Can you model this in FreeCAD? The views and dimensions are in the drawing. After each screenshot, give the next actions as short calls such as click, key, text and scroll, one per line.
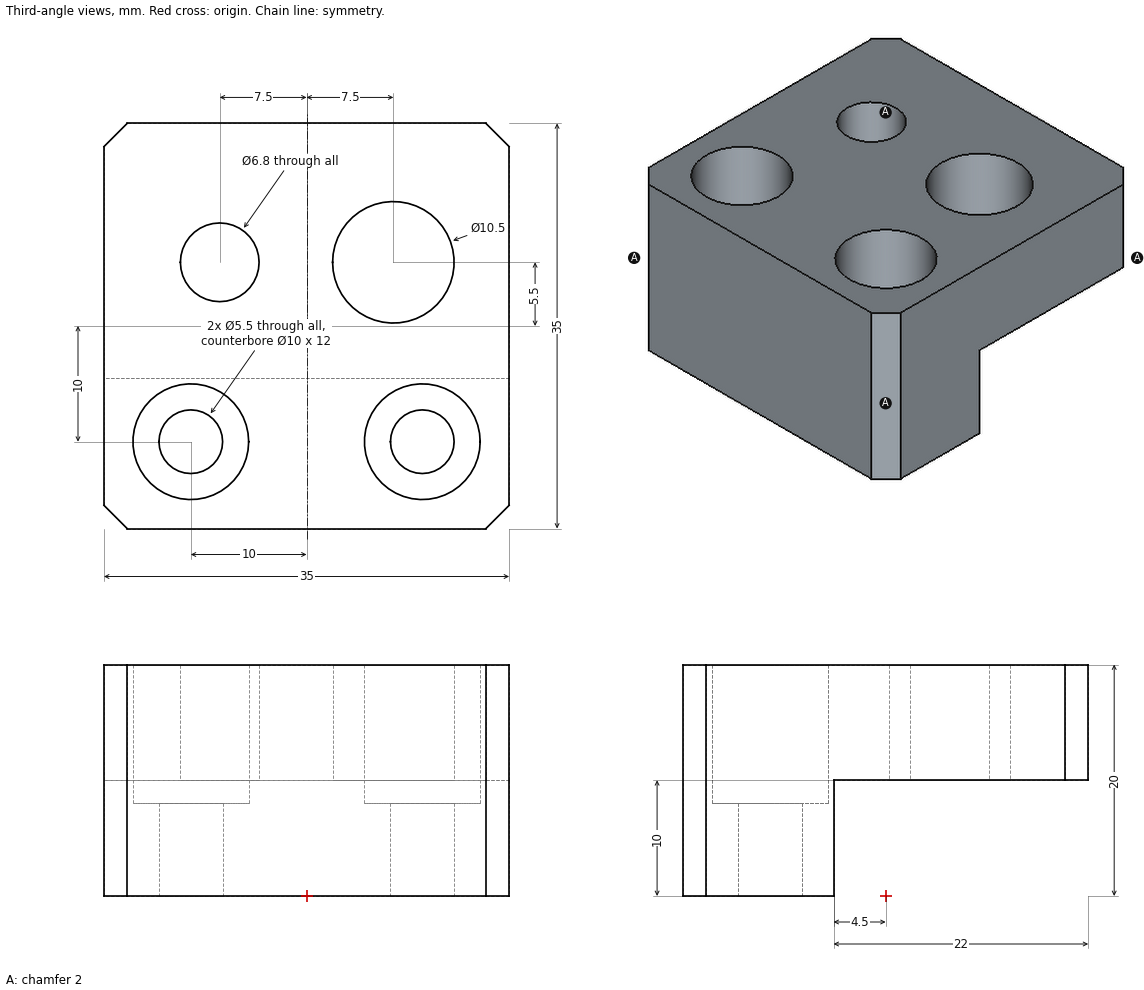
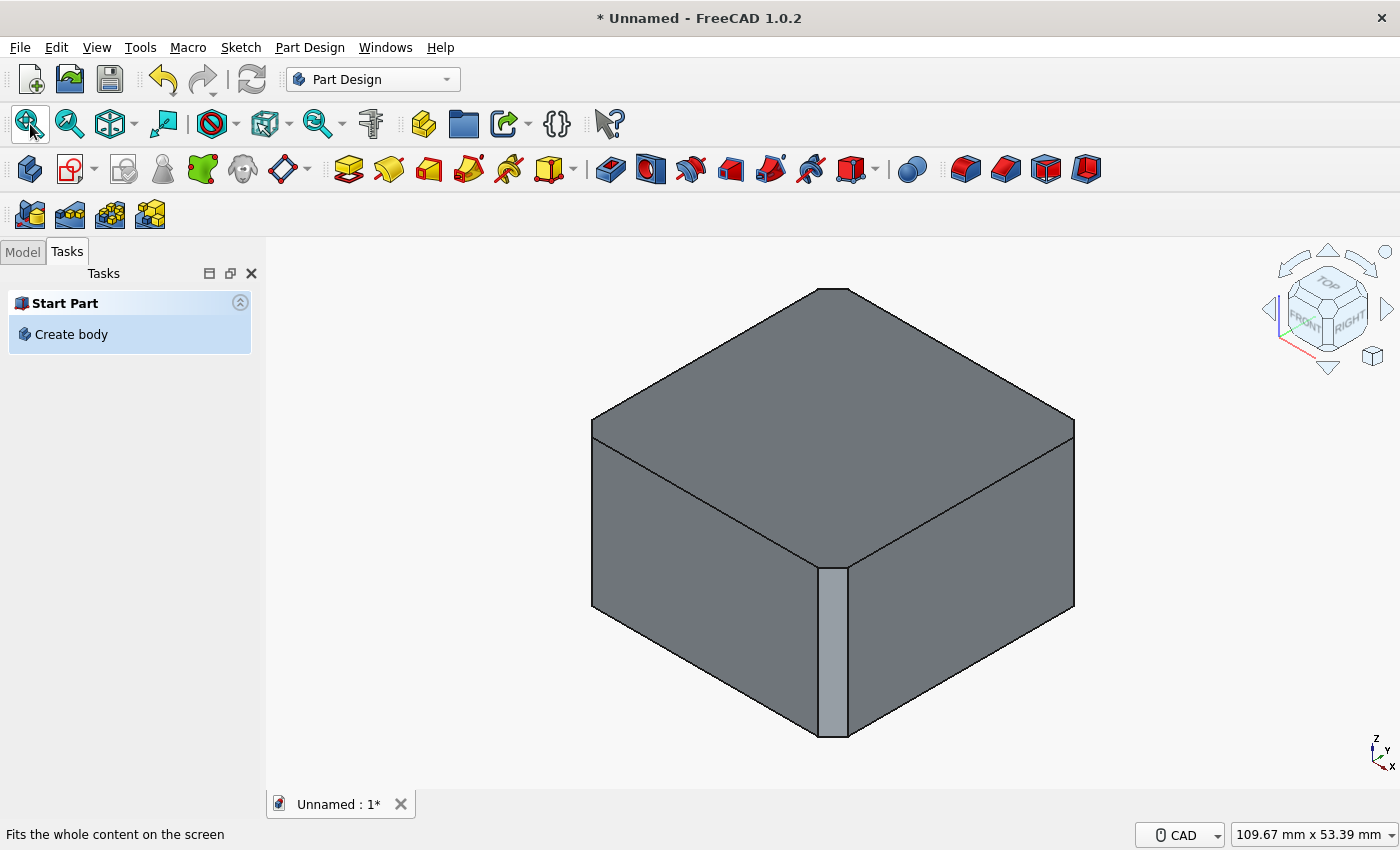
click(833, 428)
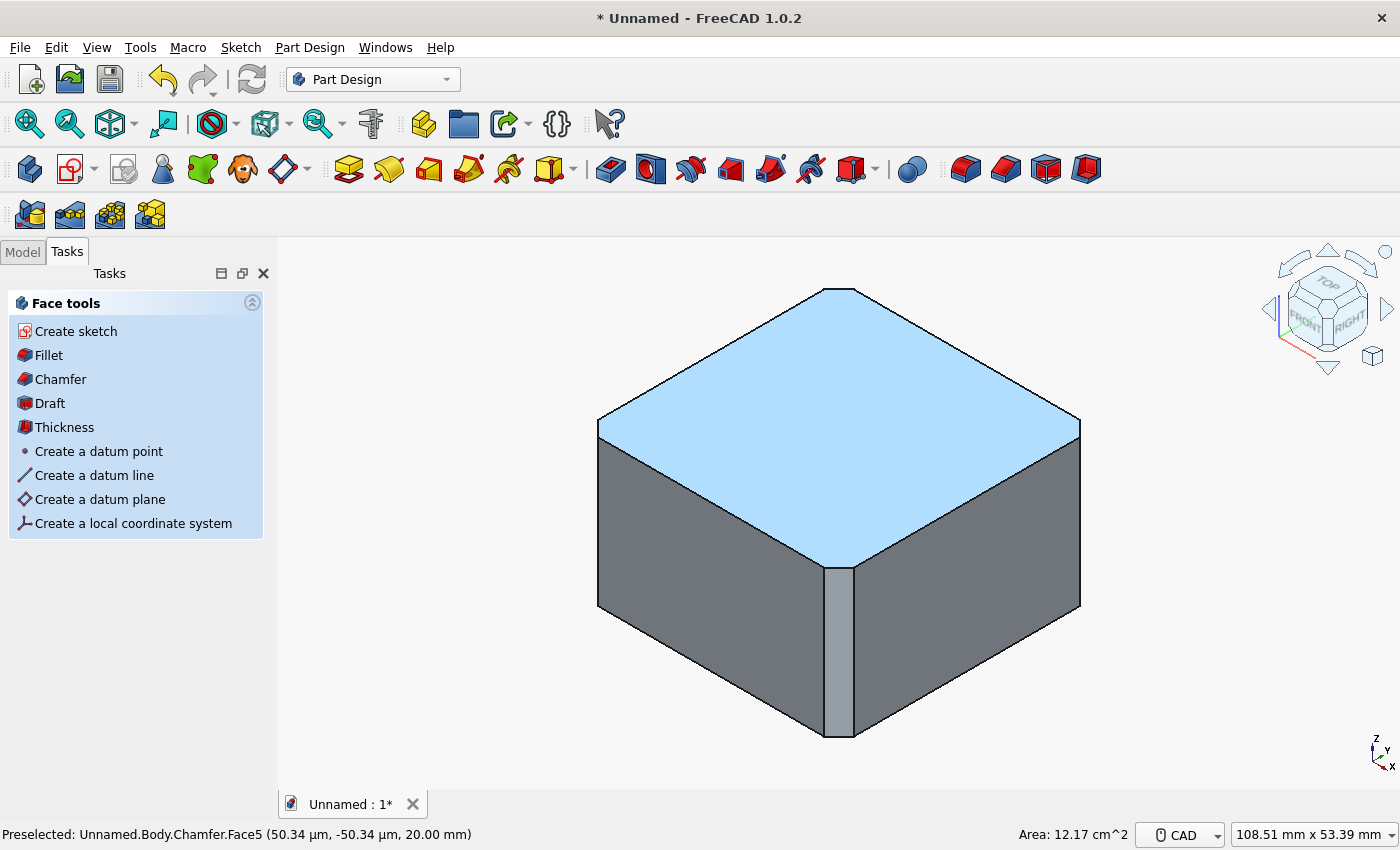
click(70, 170)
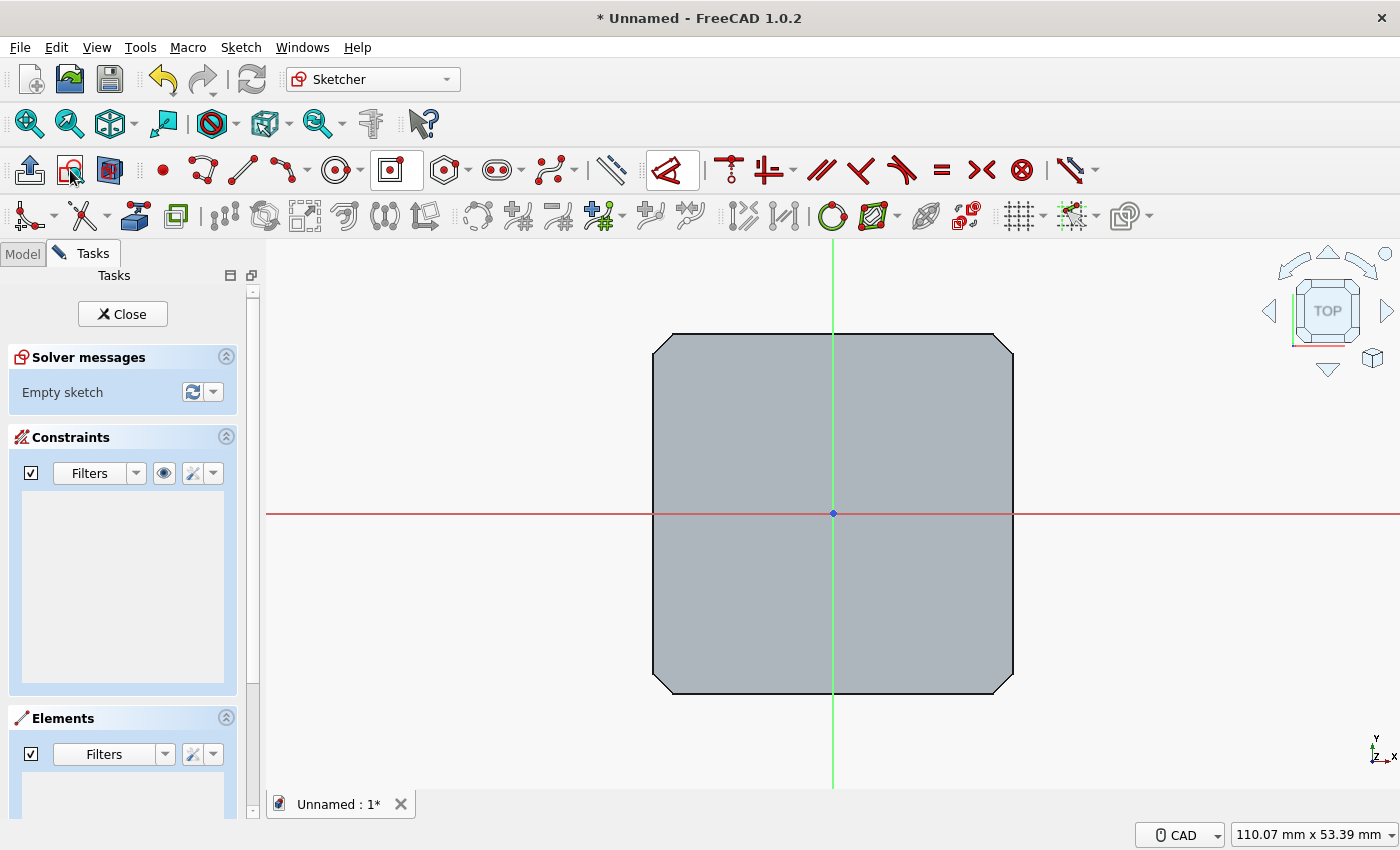
scroll(957, 435, up, 6)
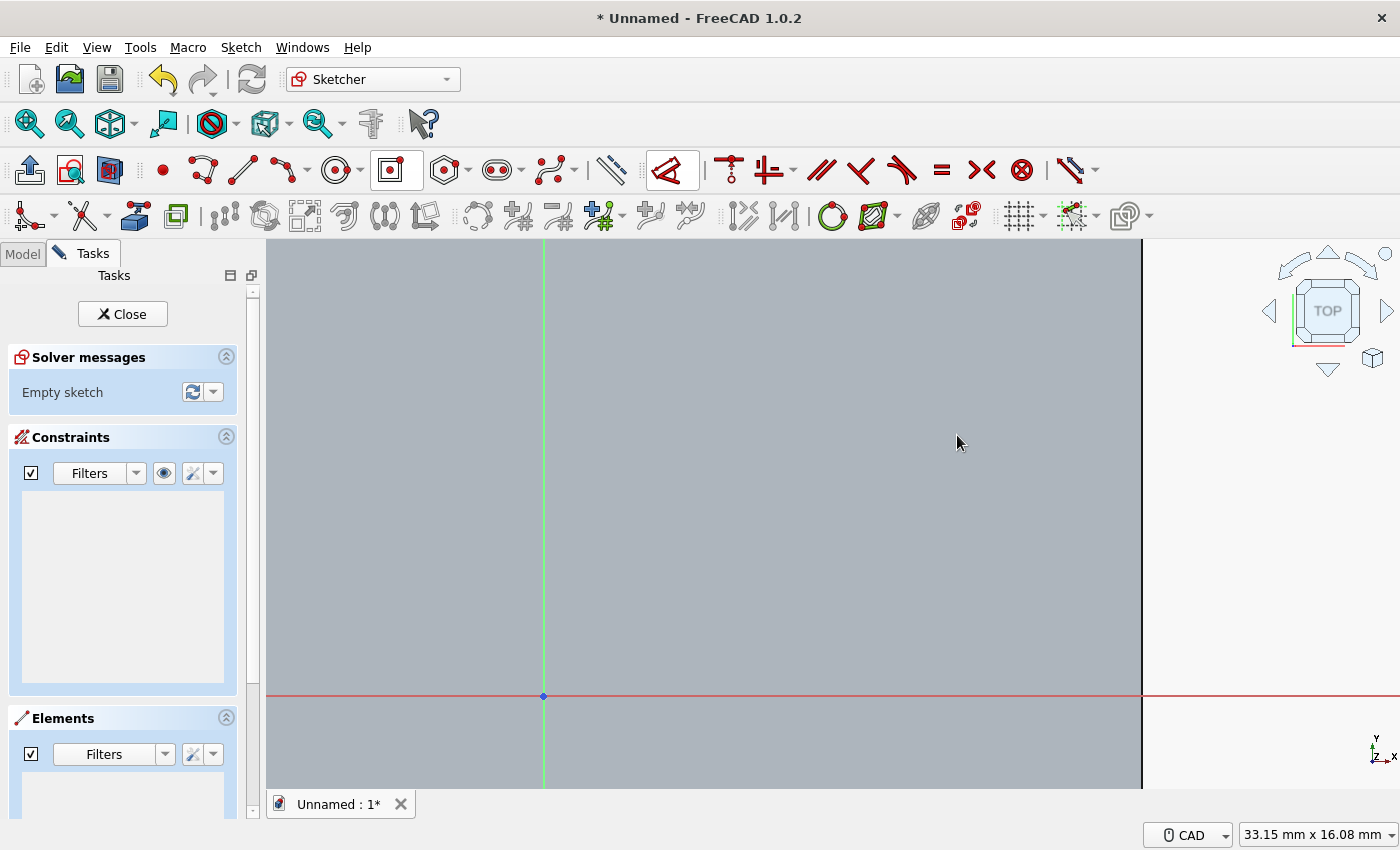
key(g)
key(c)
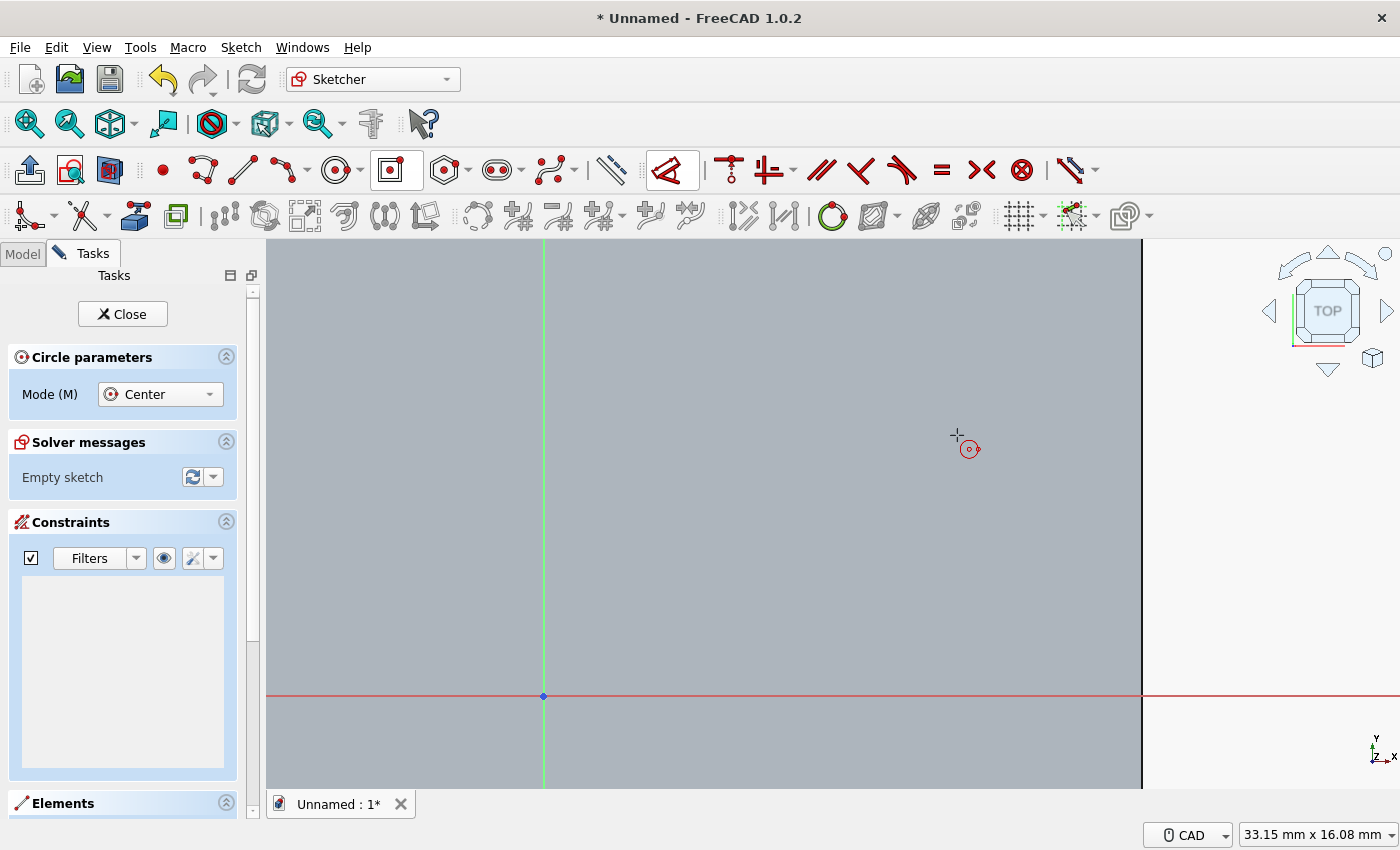
click(800, 508)
move(927, 381)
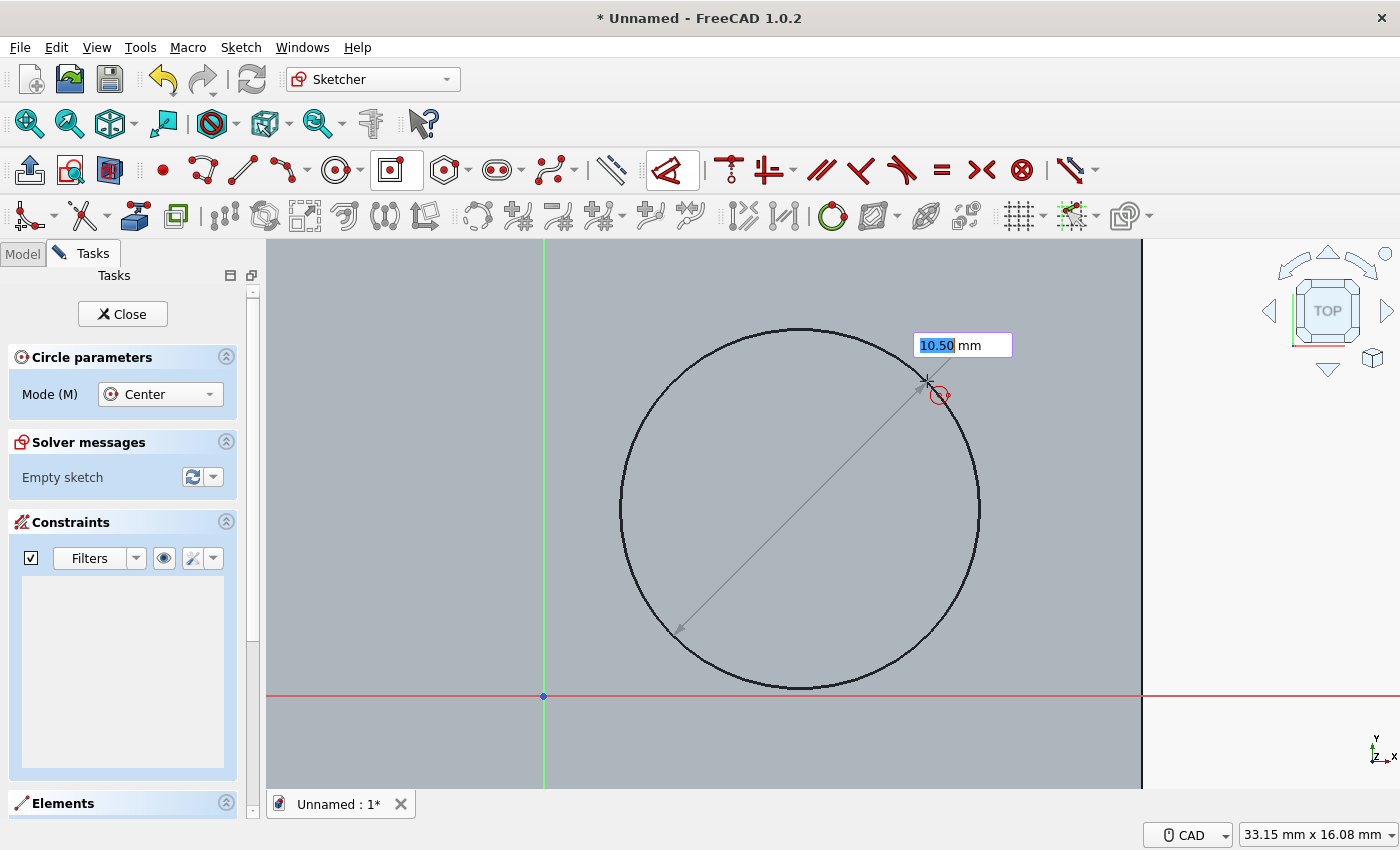
text(10.5)
key(Return)
key(Escape)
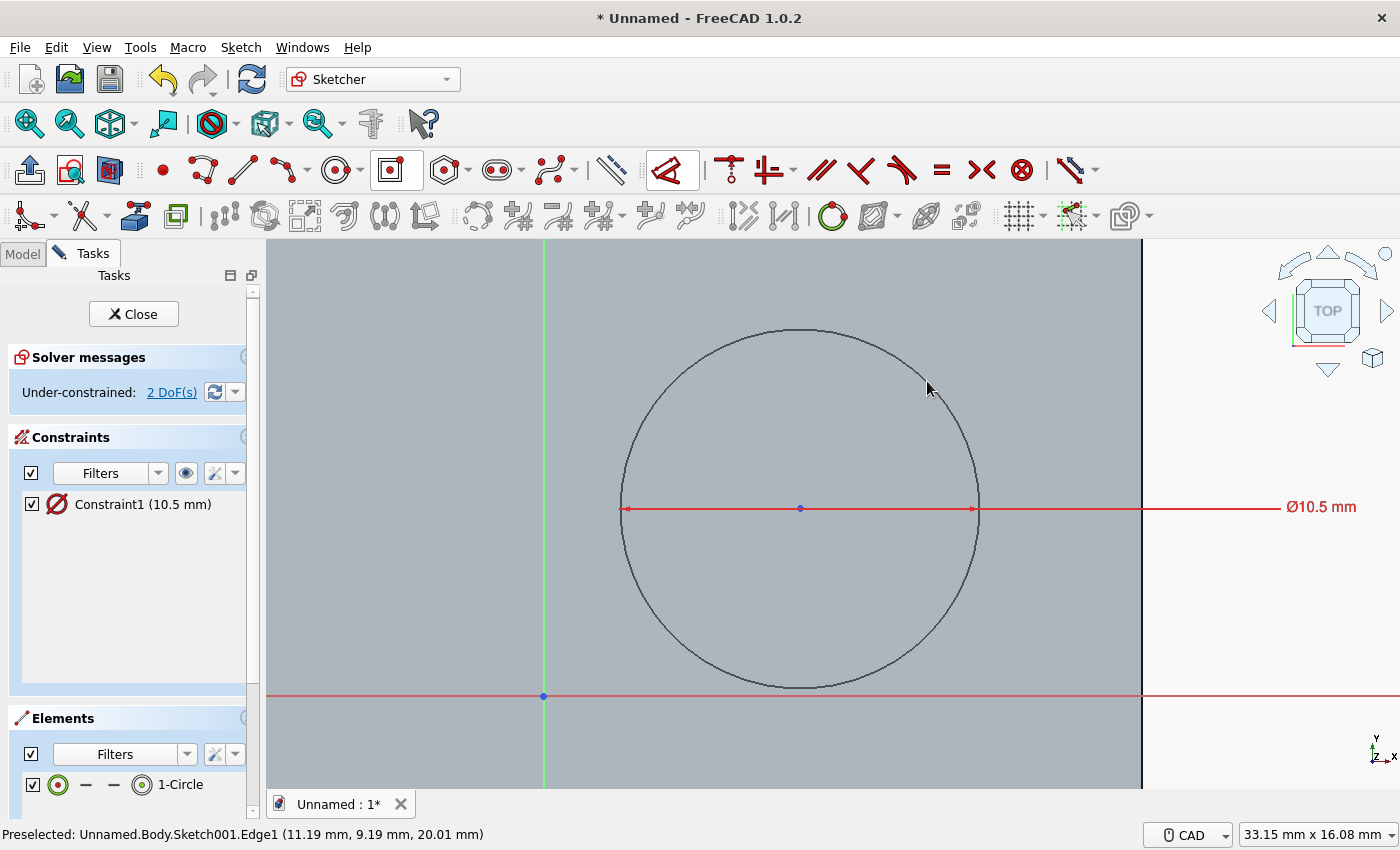
click(666, 170)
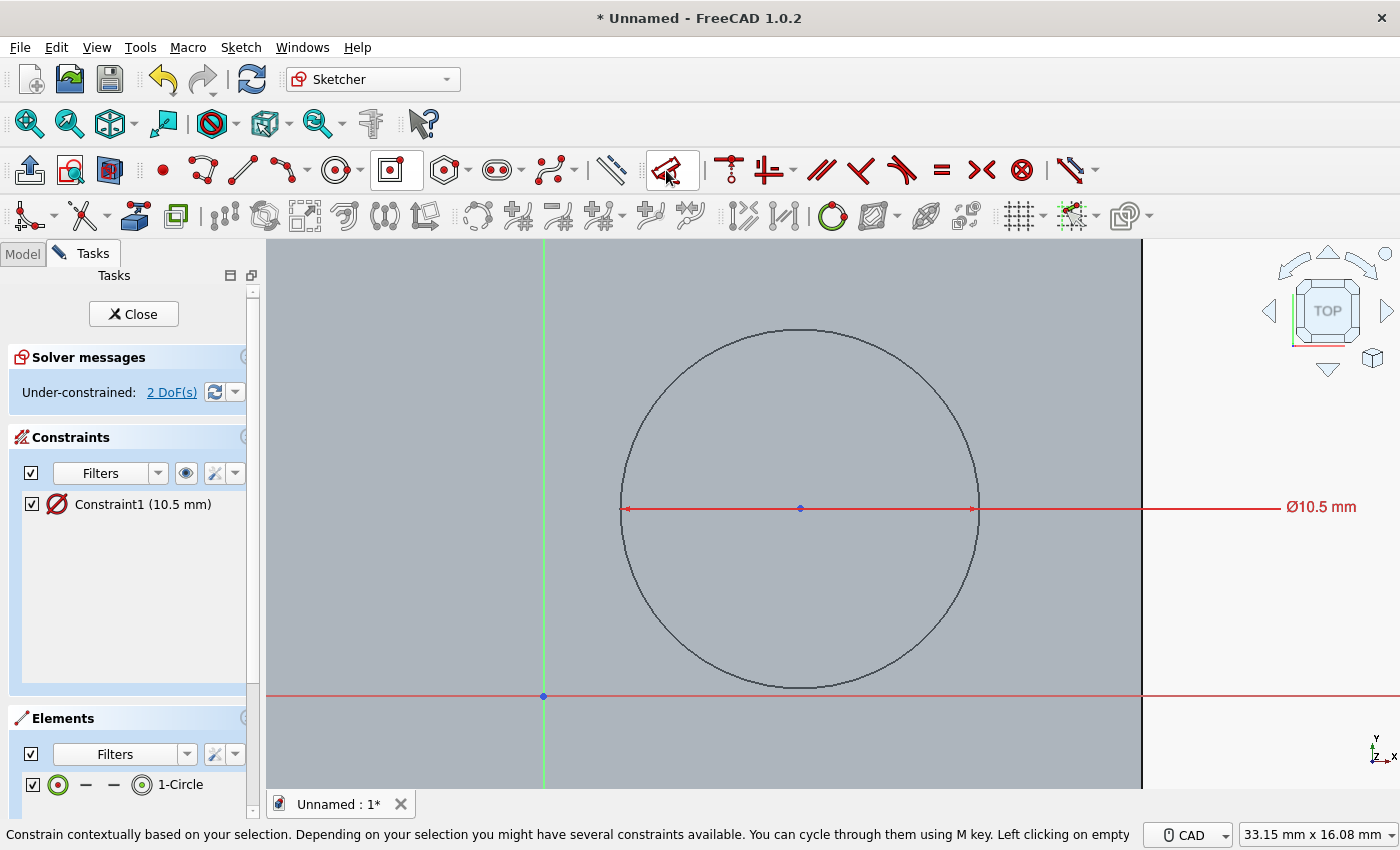
click(800, 509)
click(672, 730)